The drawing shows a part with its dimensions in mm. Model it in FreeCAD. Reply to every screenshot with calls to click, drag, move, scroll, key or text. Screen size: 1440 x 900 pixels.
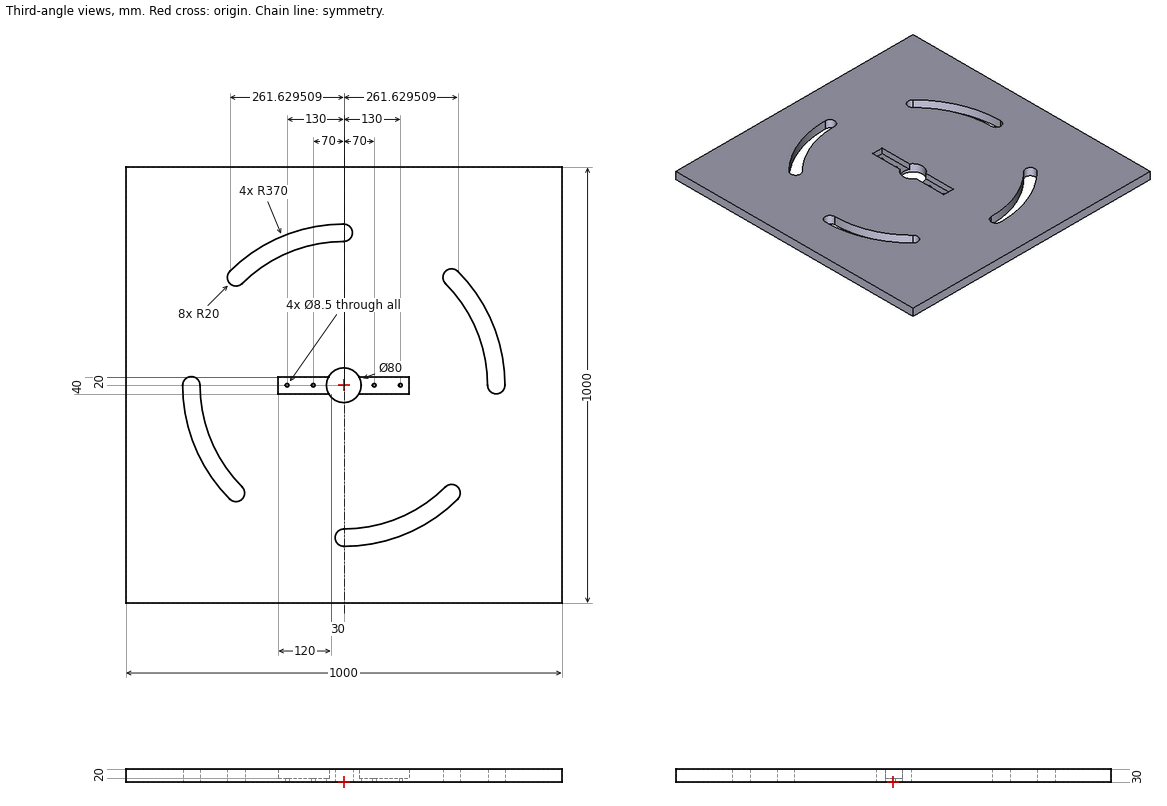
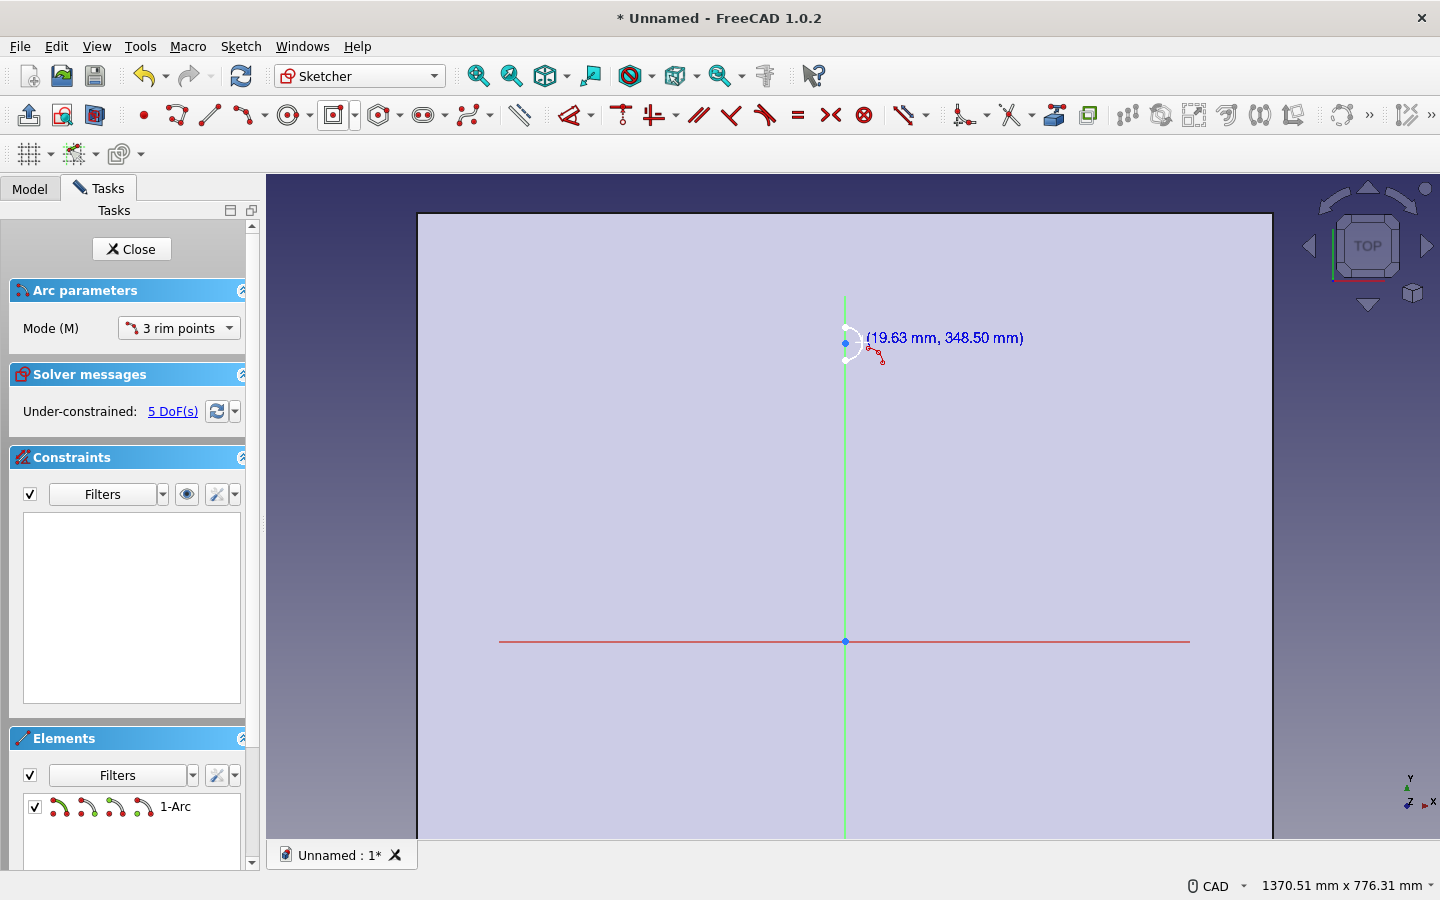
click(845, 327)
click(621, 417)
click(724, 349)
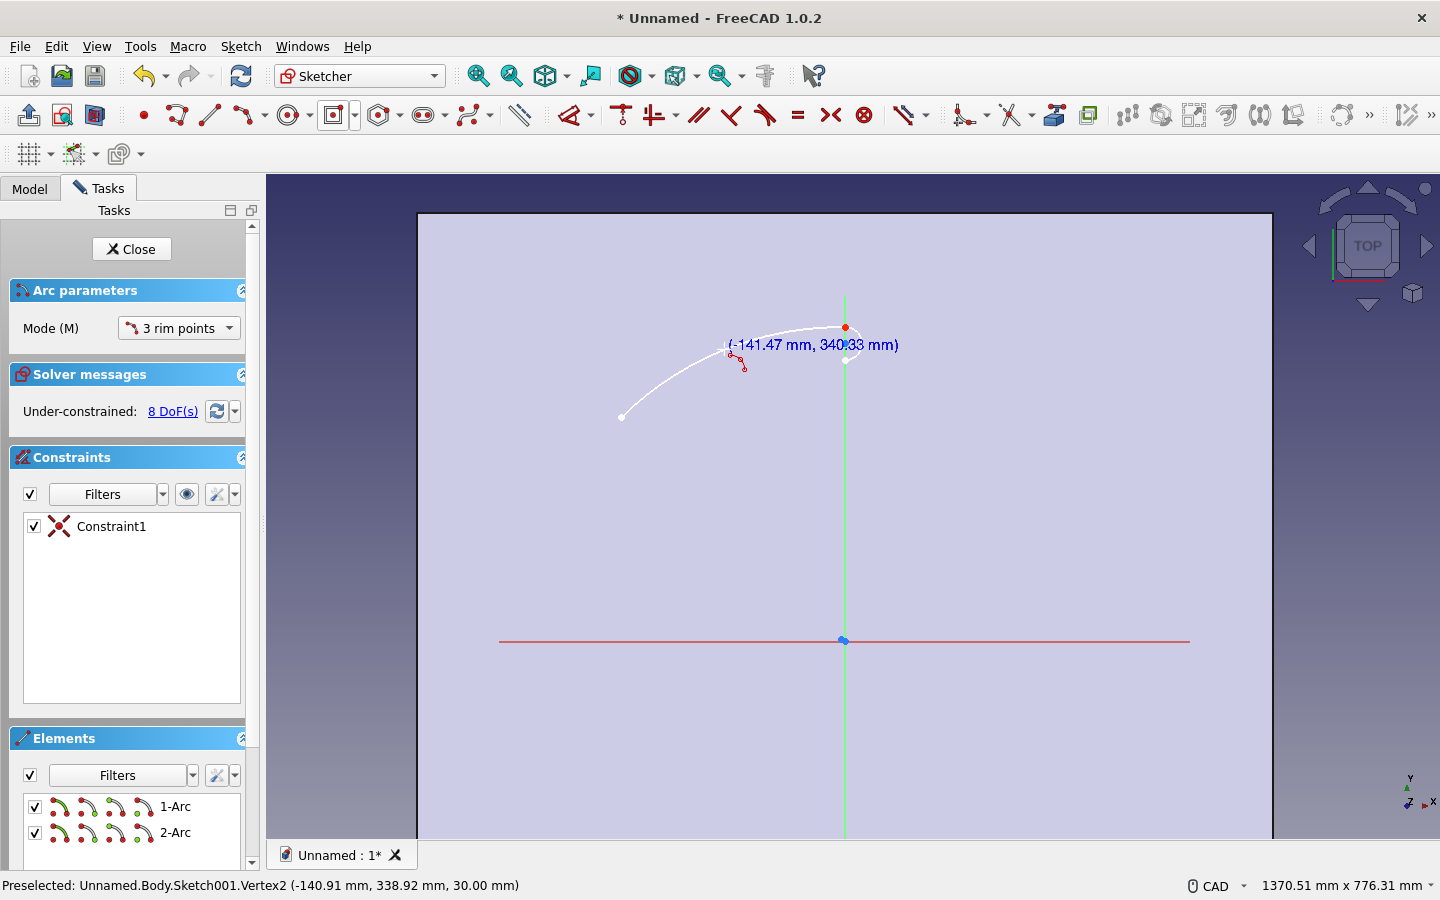
click(621, 418)
click(645, 442)
click(621, 442)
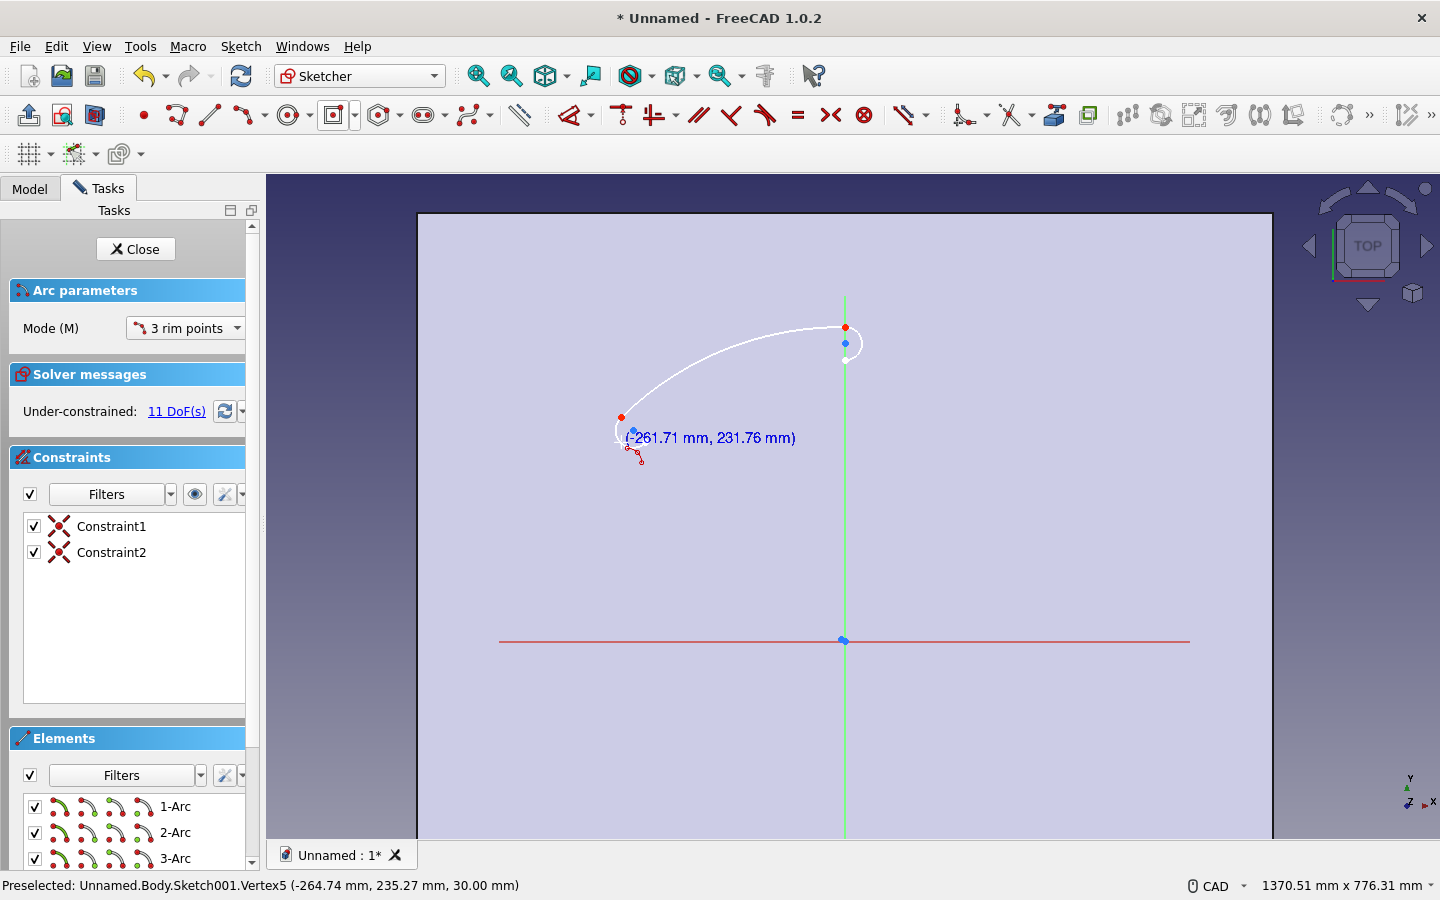
click(645, 443)
click(845, 360)
click(737, 380)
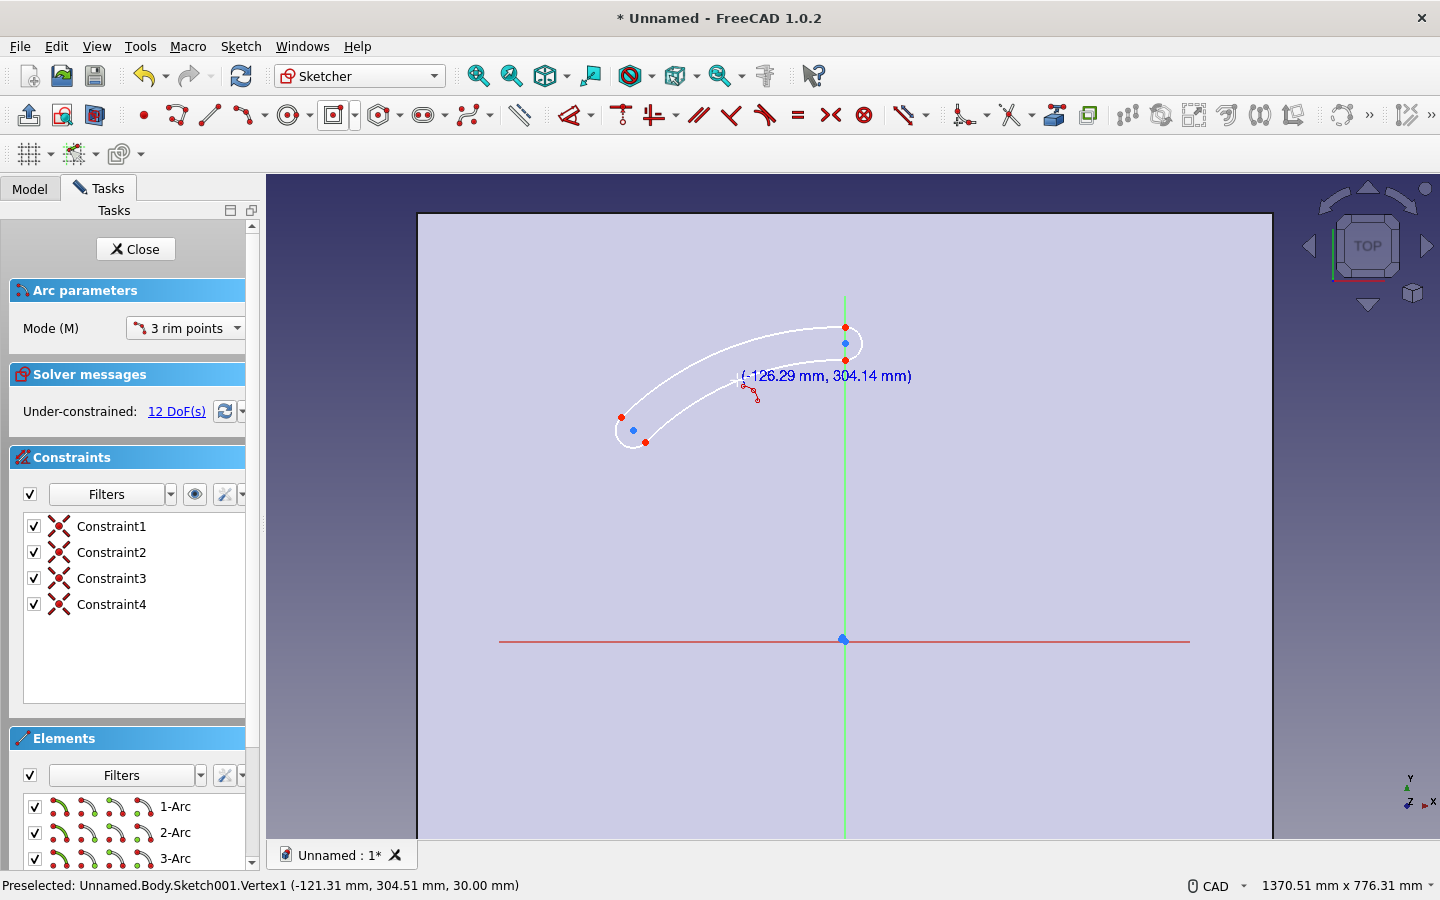
click(1128, 642)
click(1162, 642)
click(1145, 659)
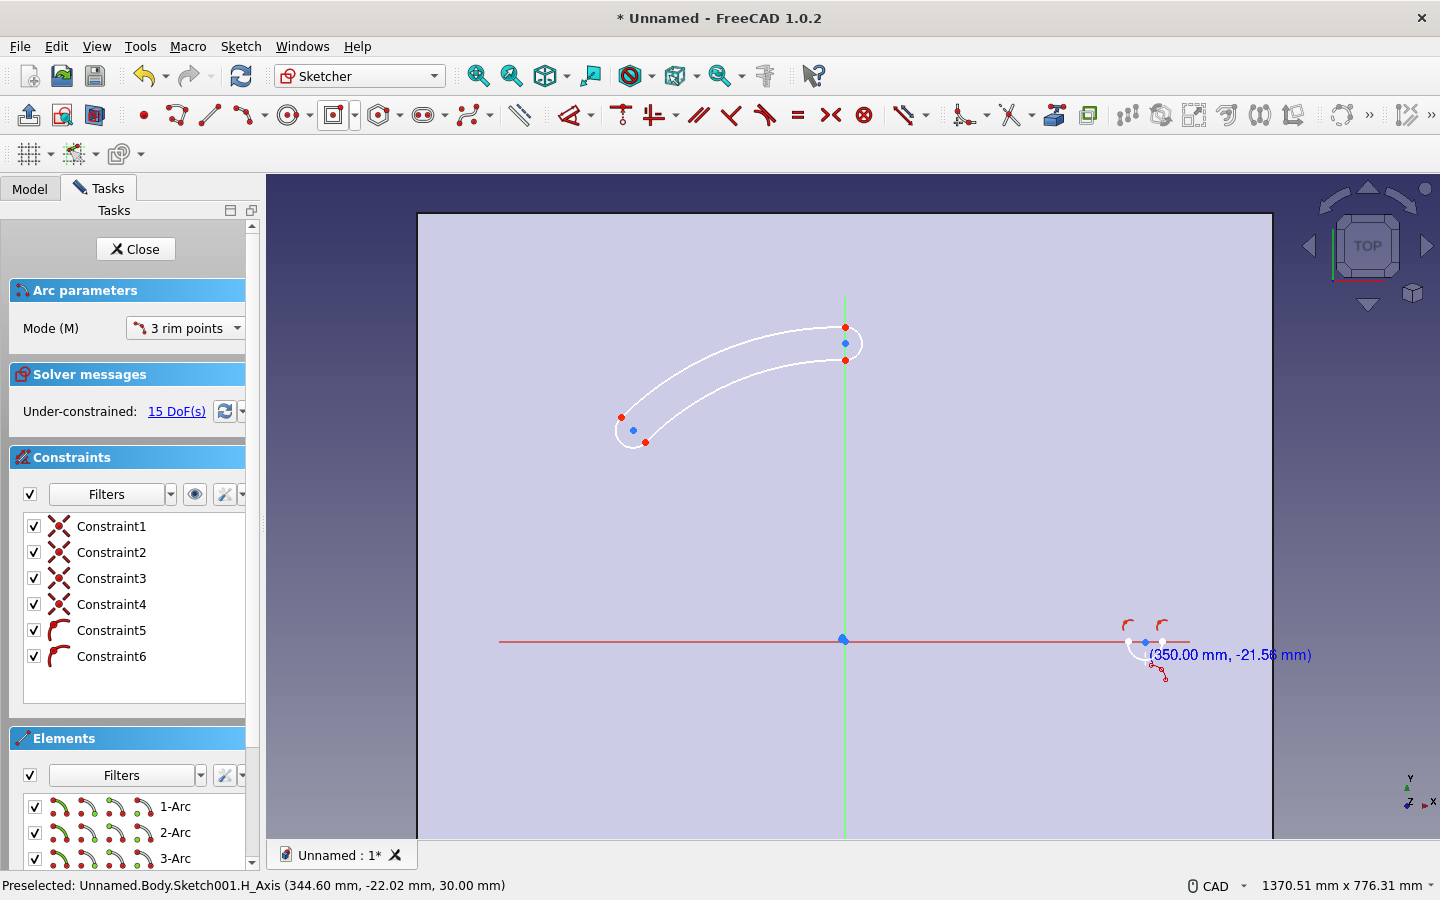
click(1162, 642)
click(1069, 417)
click(1138, 520)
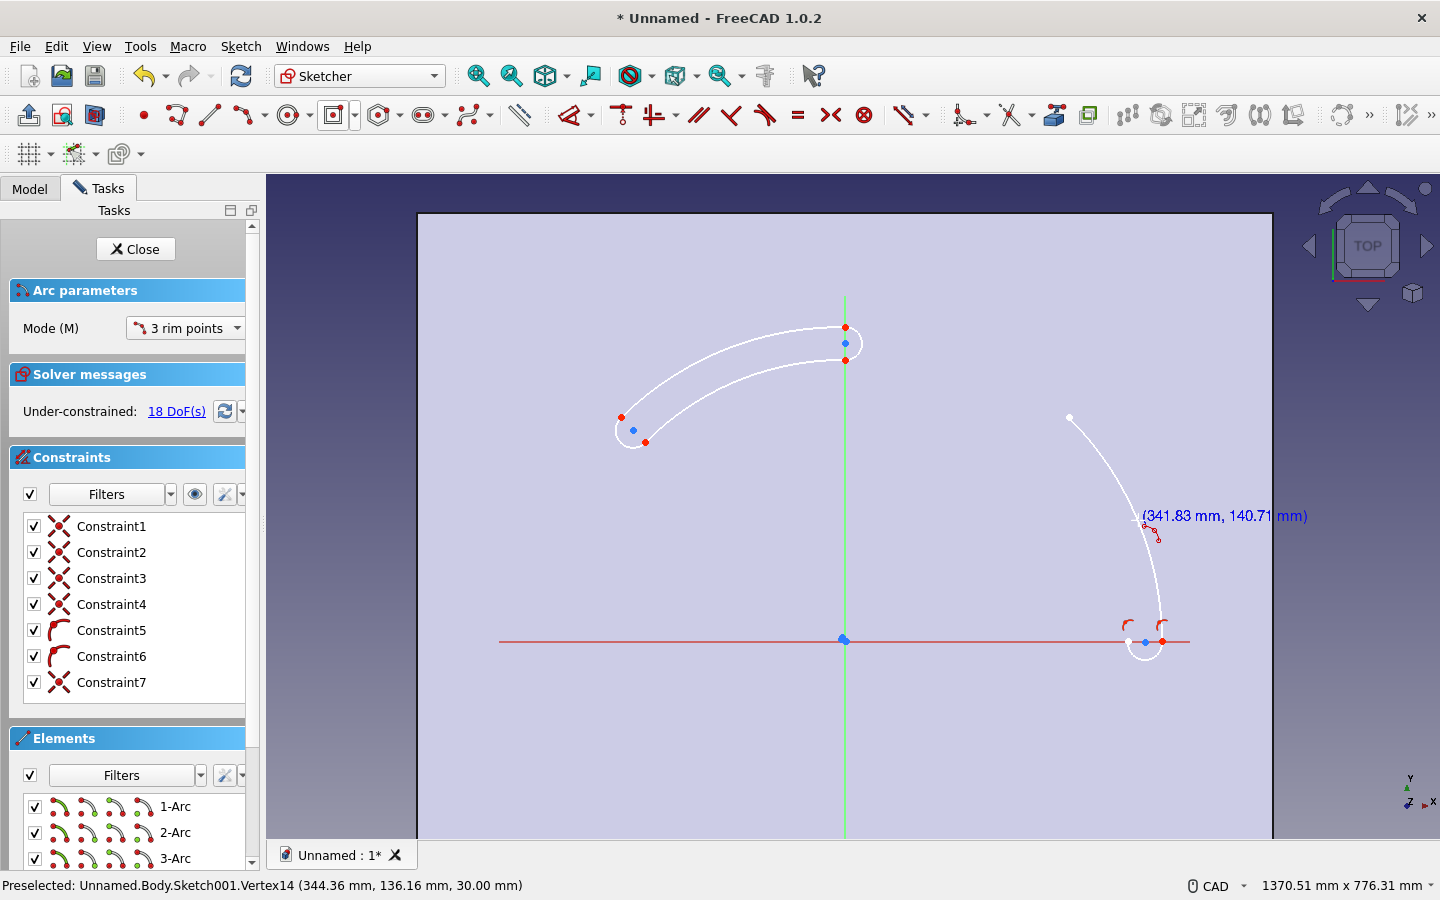
click(1069, 418)
click(1045, 442)
click(1045, 417)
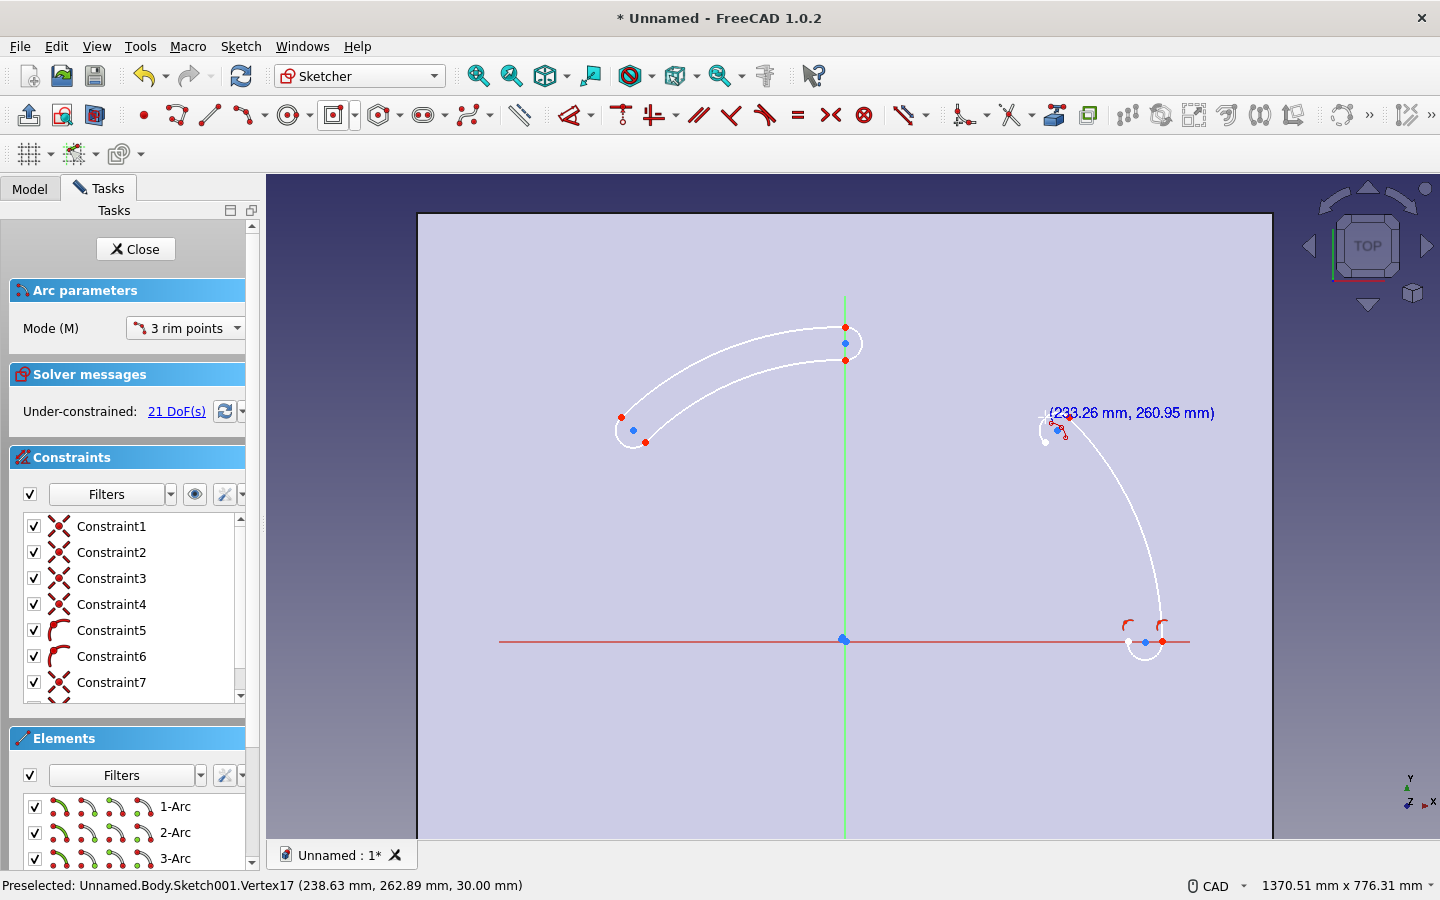
click(1045, 443)
click(1128, 642)
click(1106, 533)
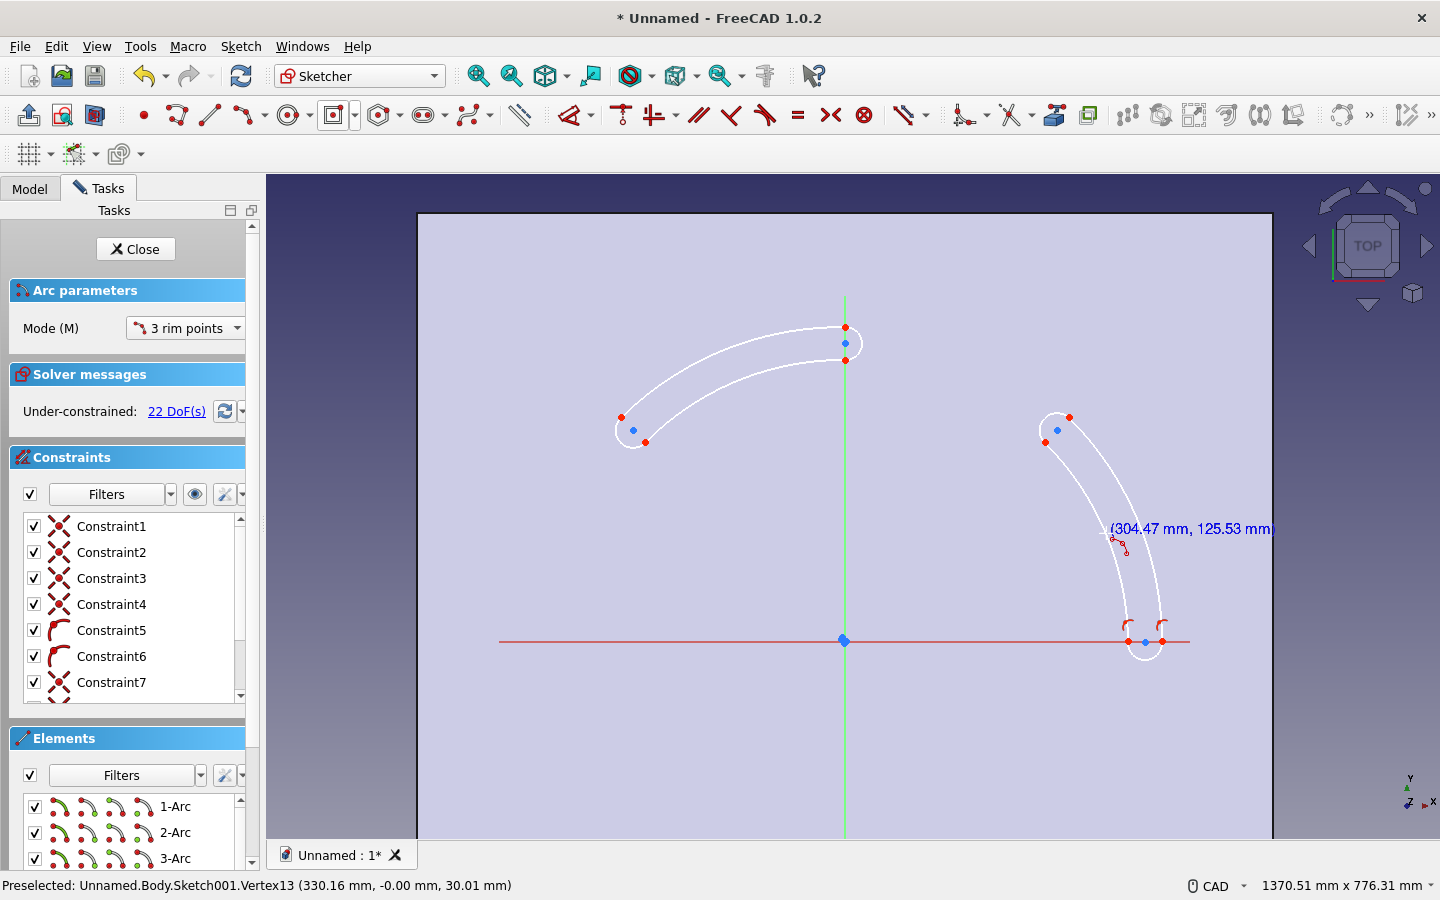
scroll(661, 232, down, 2)